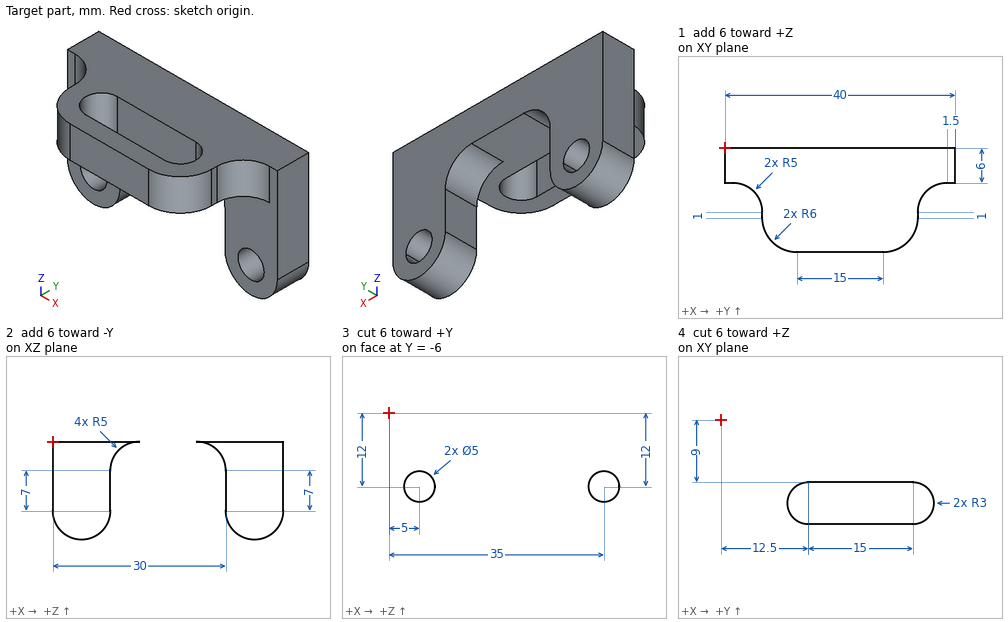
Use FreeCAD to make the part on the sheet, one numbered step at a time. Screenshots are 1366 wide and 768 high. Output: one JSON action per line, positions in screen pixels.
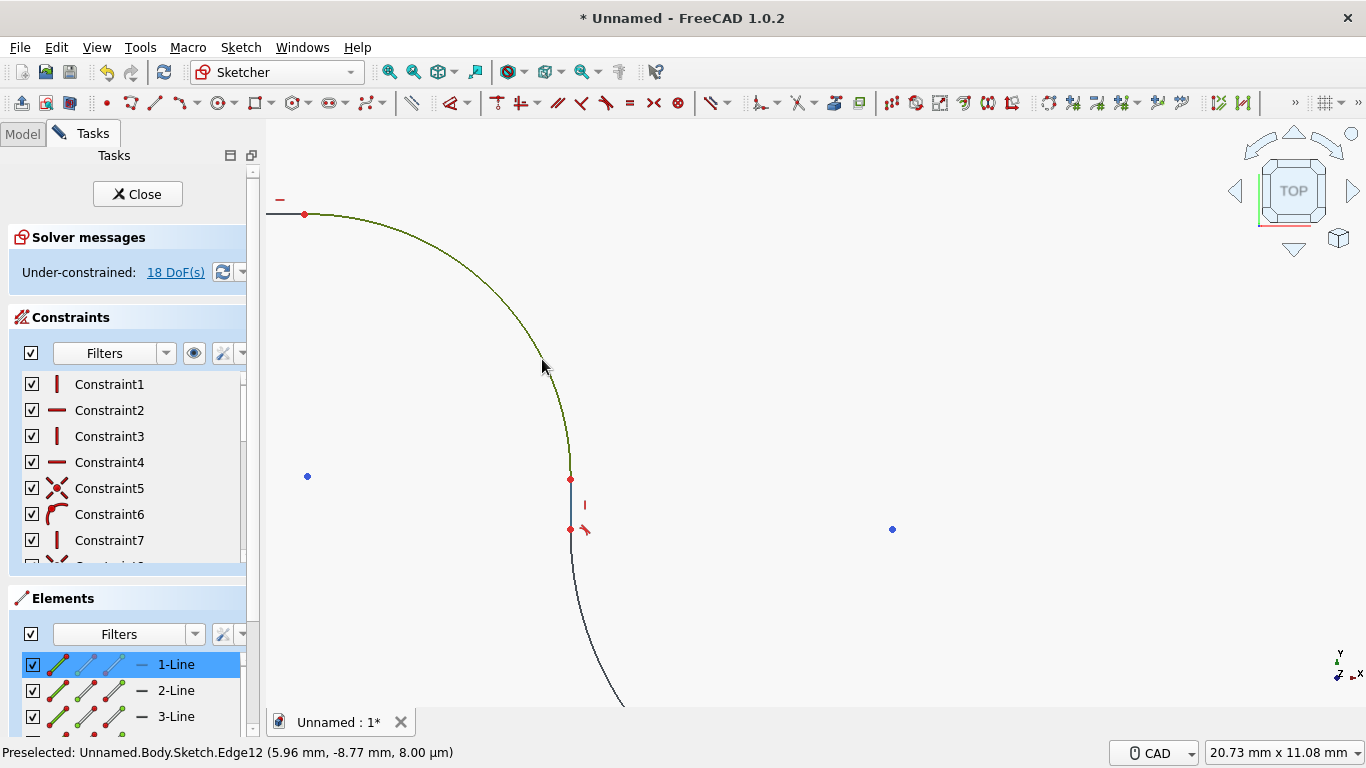
{"action": "key", "text": "t"}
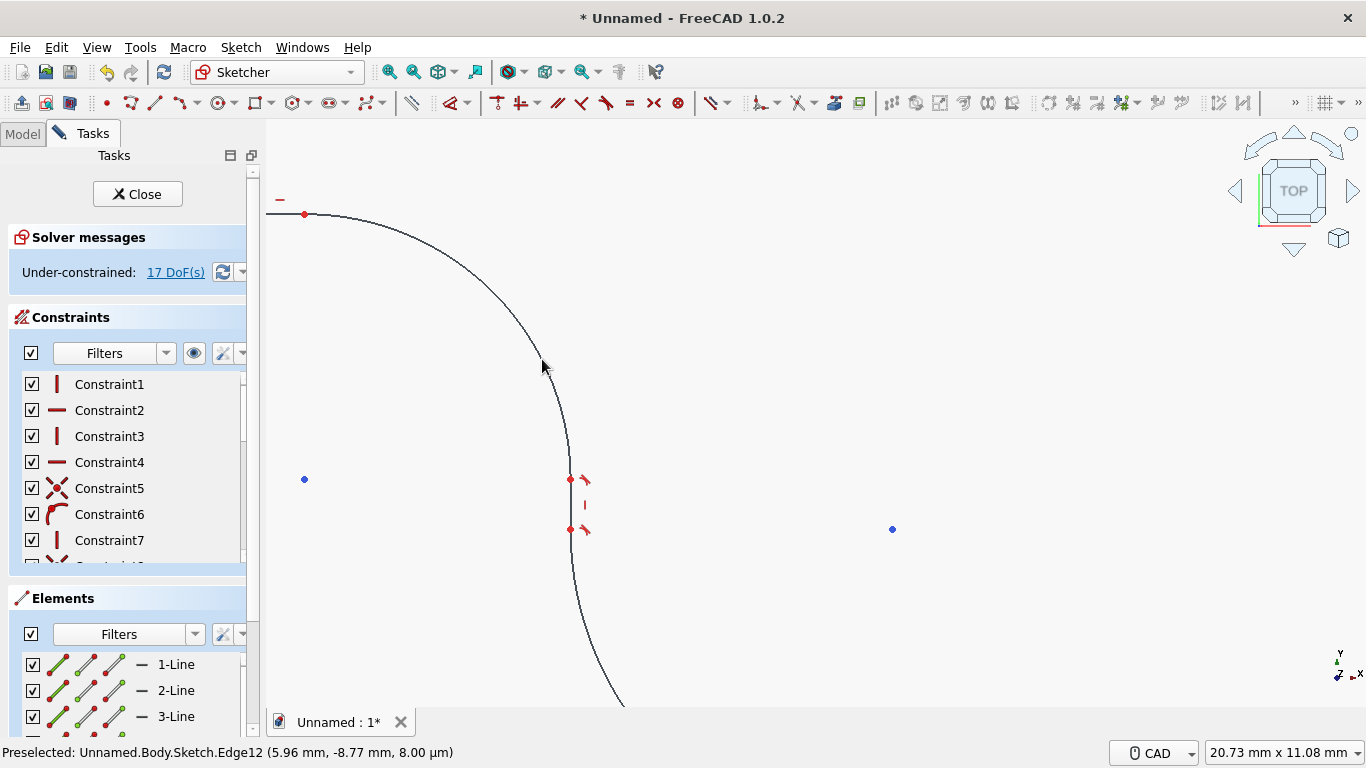
{"action": "scroll", "coordinate": [514, 431], "scroll_direction": "down", "scroll_amount": 6}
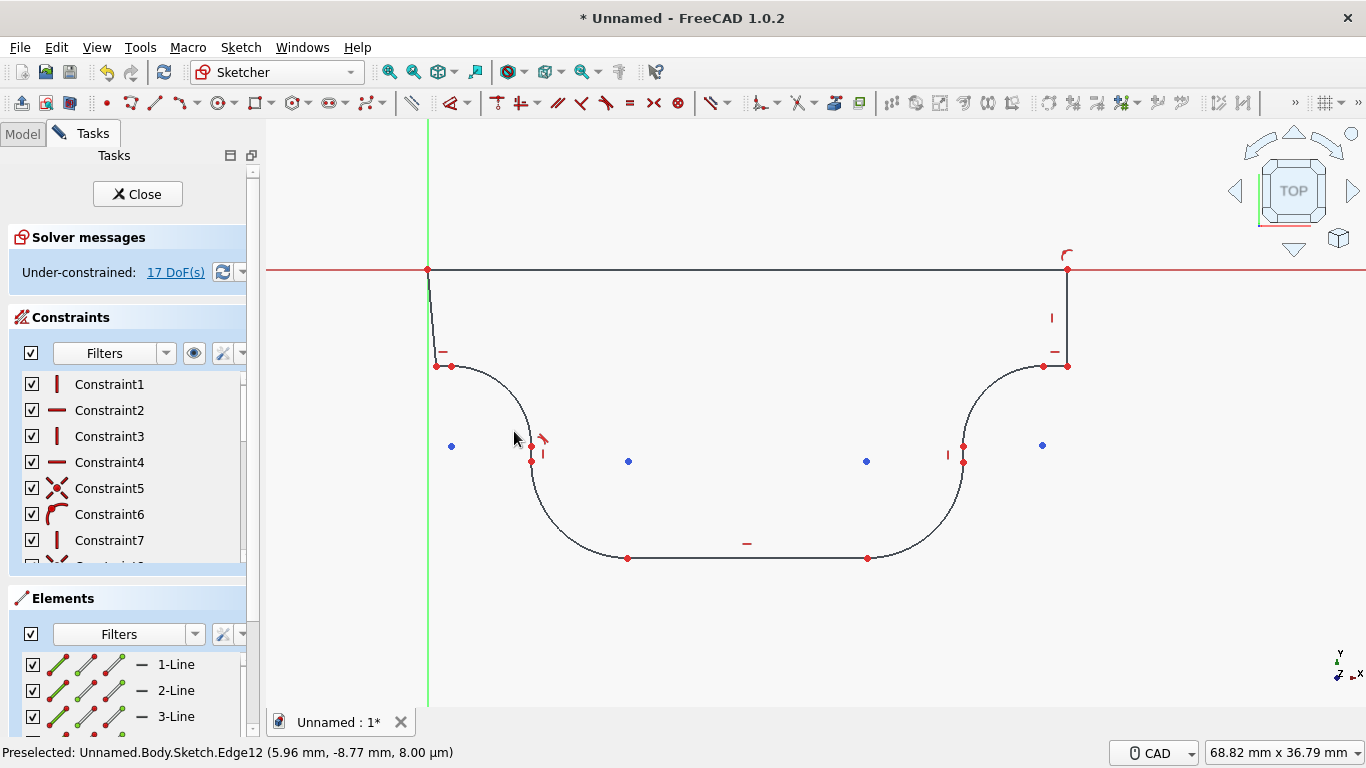
{"action": "left_click", "coordinate": [699, 558]}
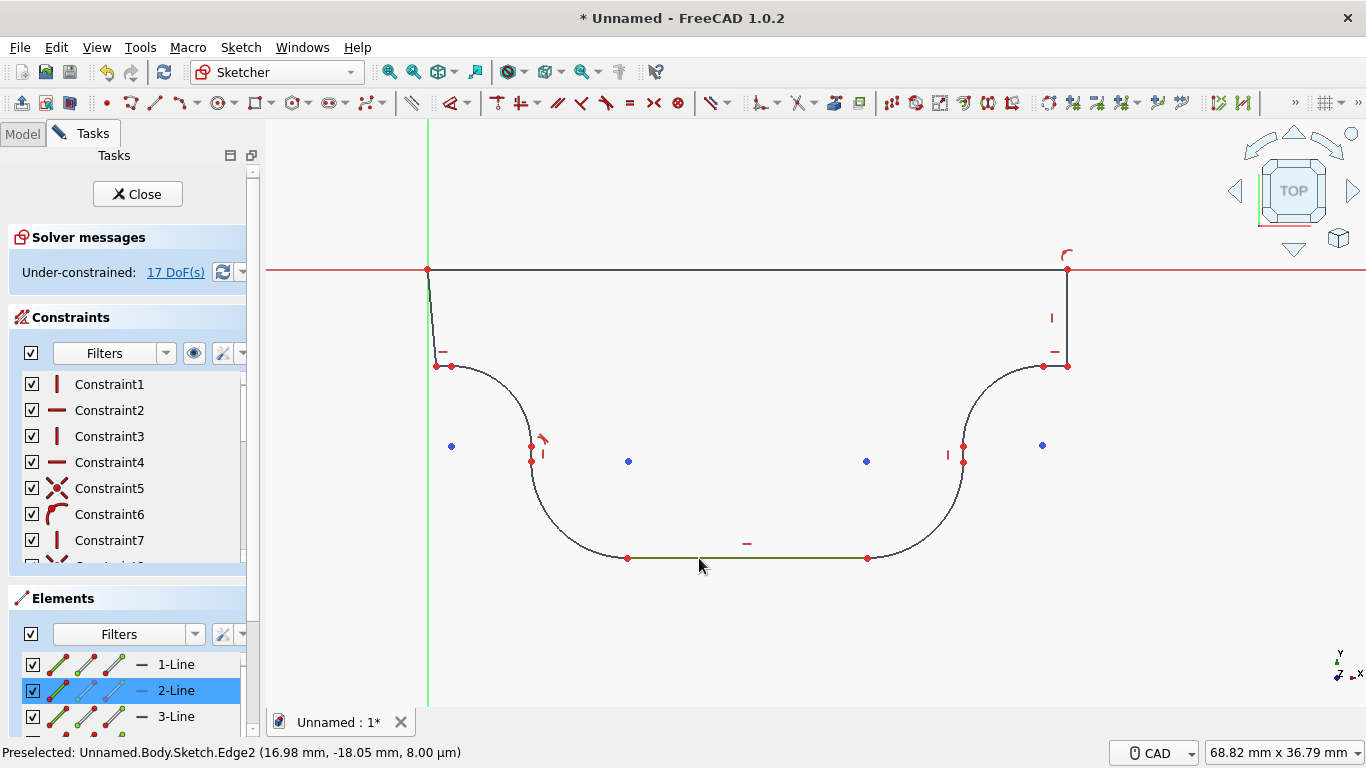
{"action": "left_click", "coordinate": [542, 505]}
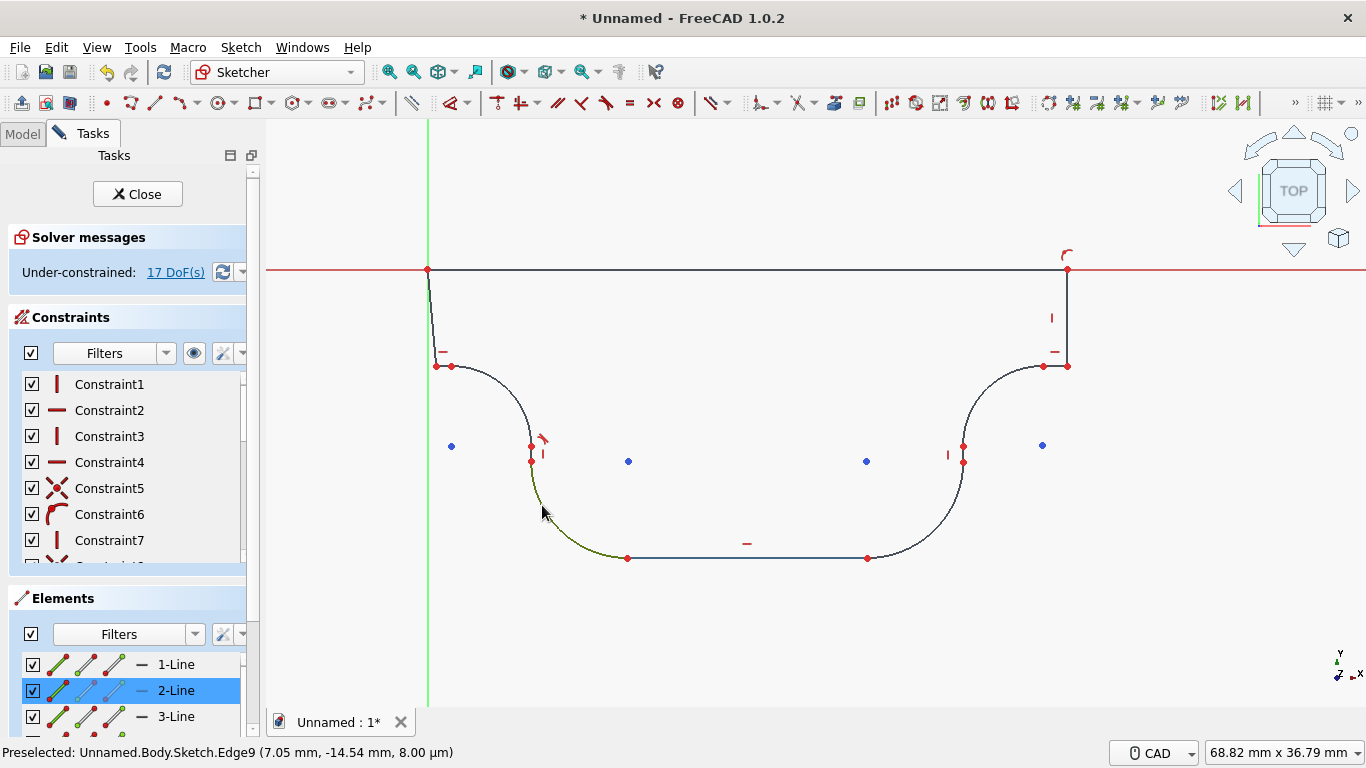
{"action": "key", "text": "t"}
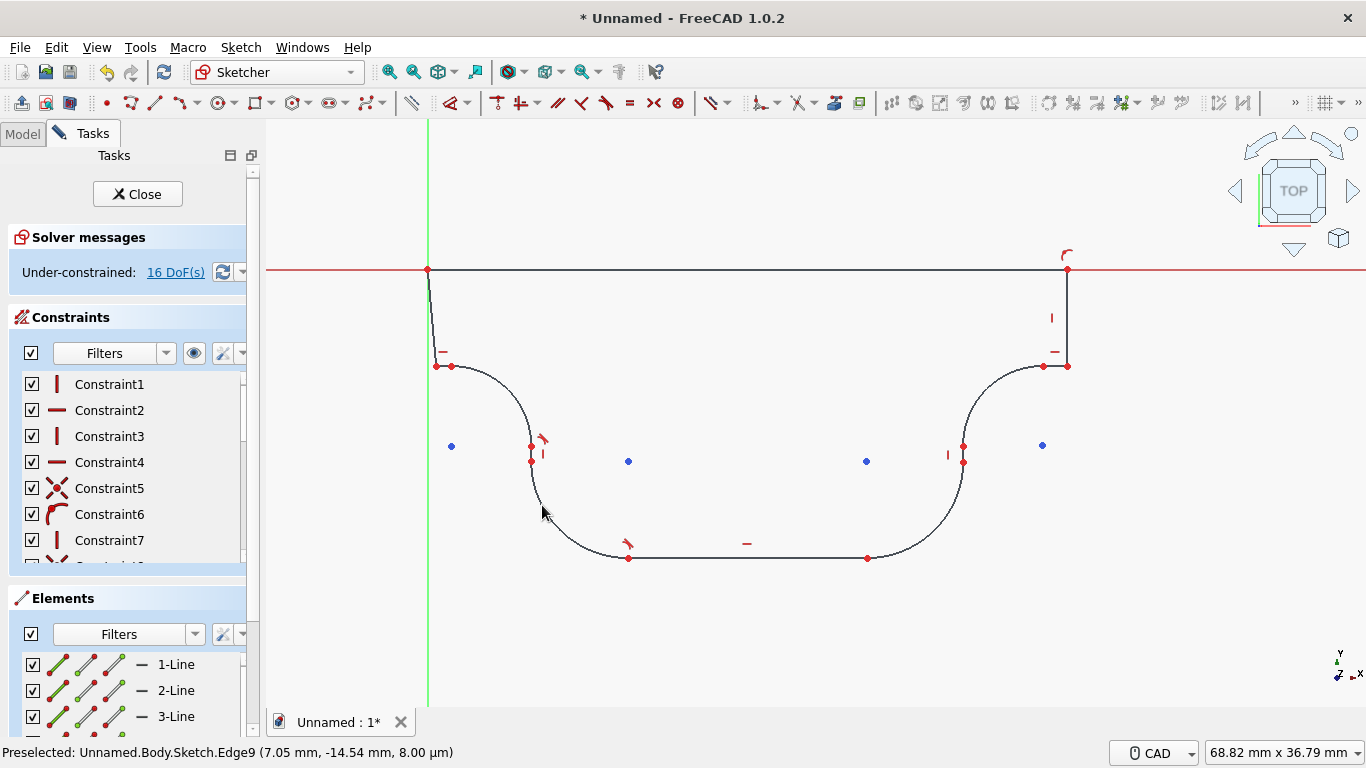
{"action": "left_click", "coordinate": [700, 558]}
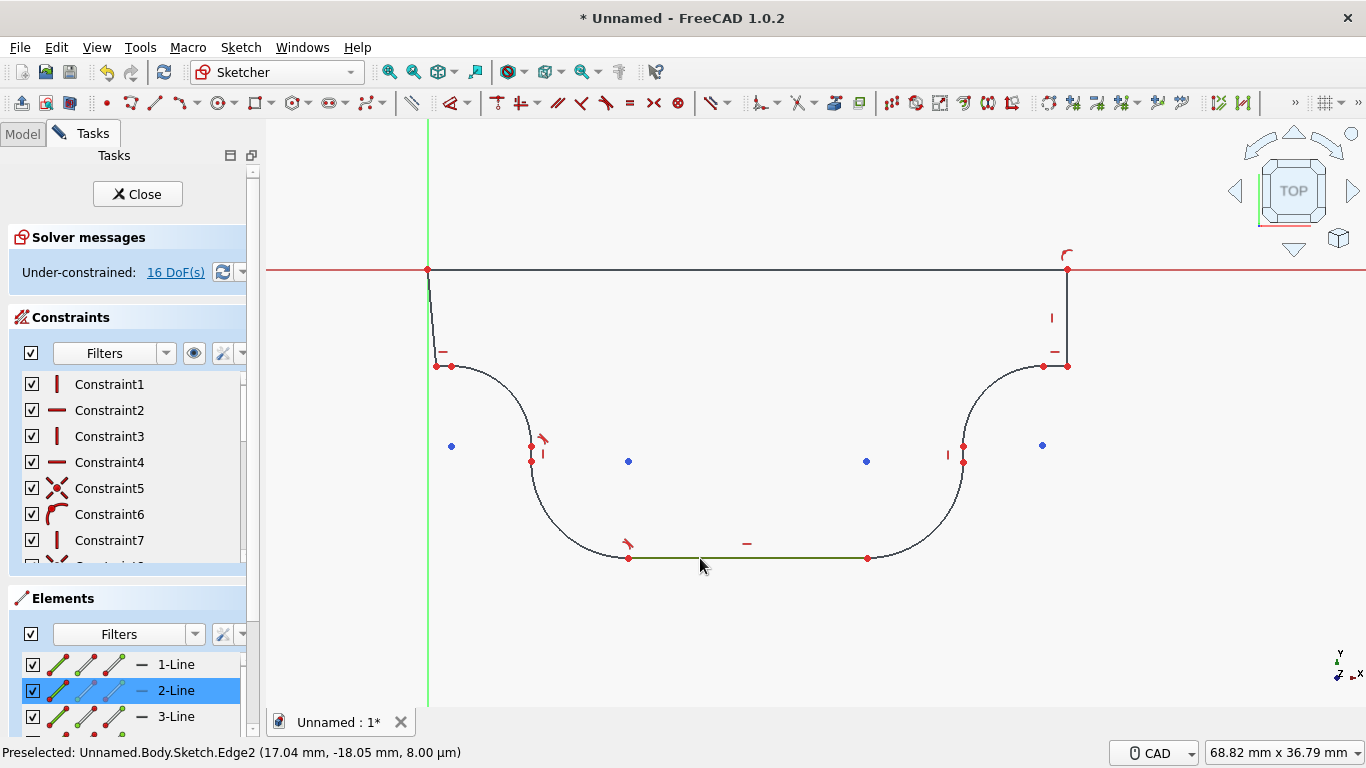
{"action": "left_click", "coordinate": [911, 547]}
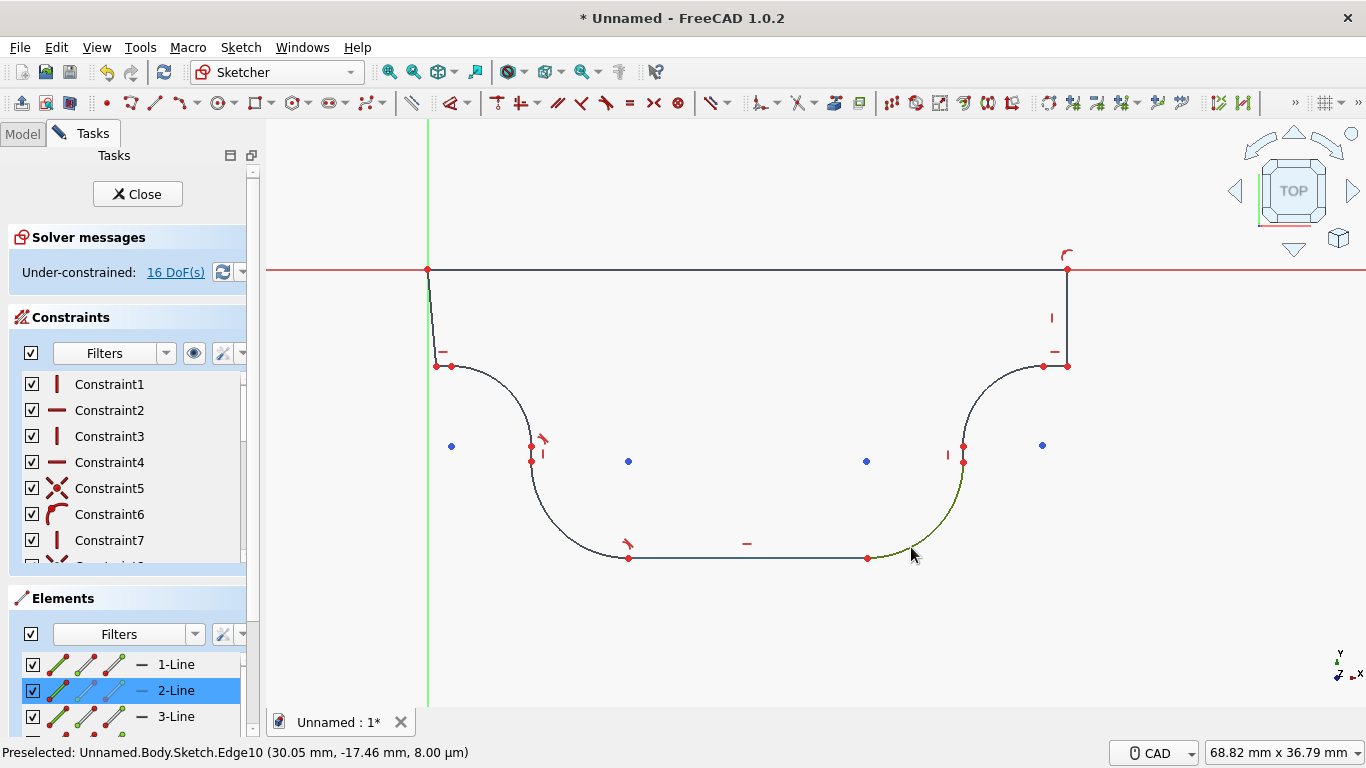
{"action": "left_click", "coordinate": [606, 104]}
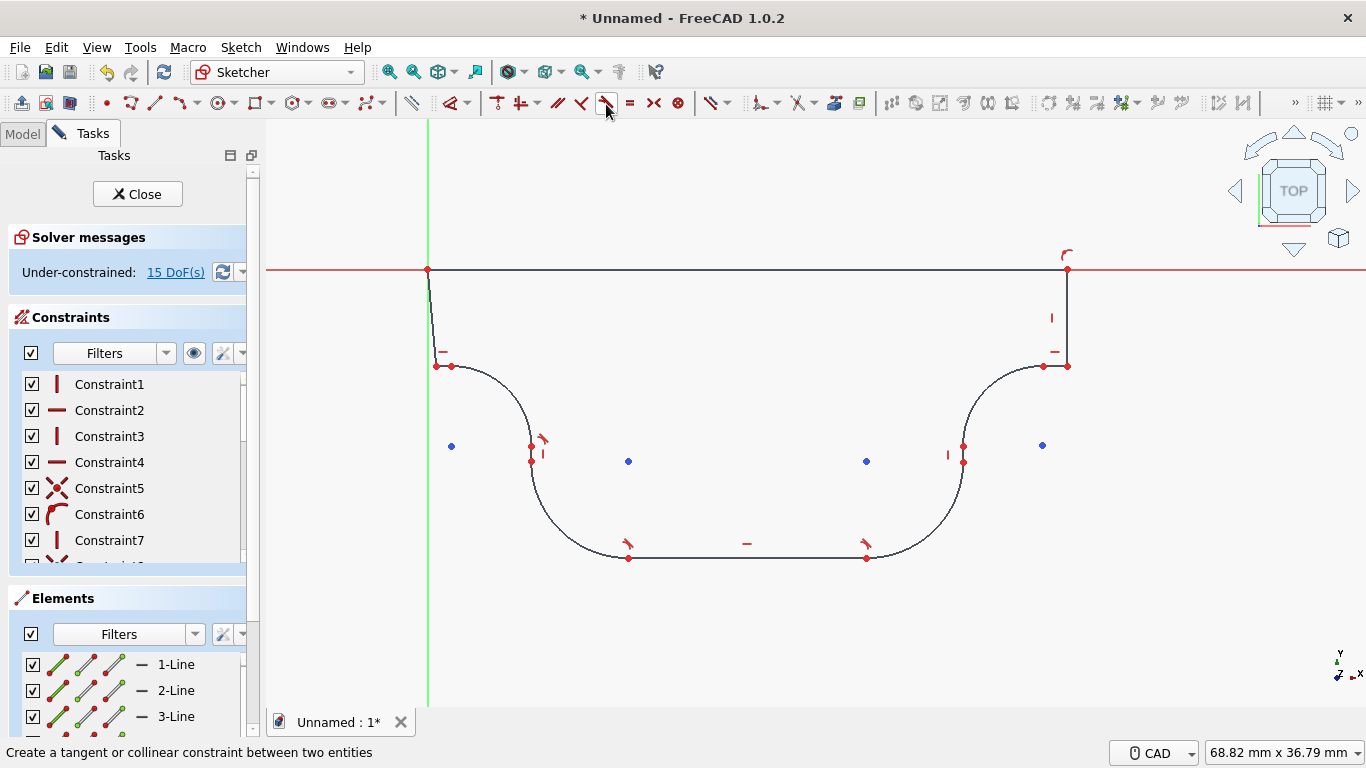
{"action": "scroll", "coordinate": [963, 454], "scroll_direction": "up", "scroll_amount": 3}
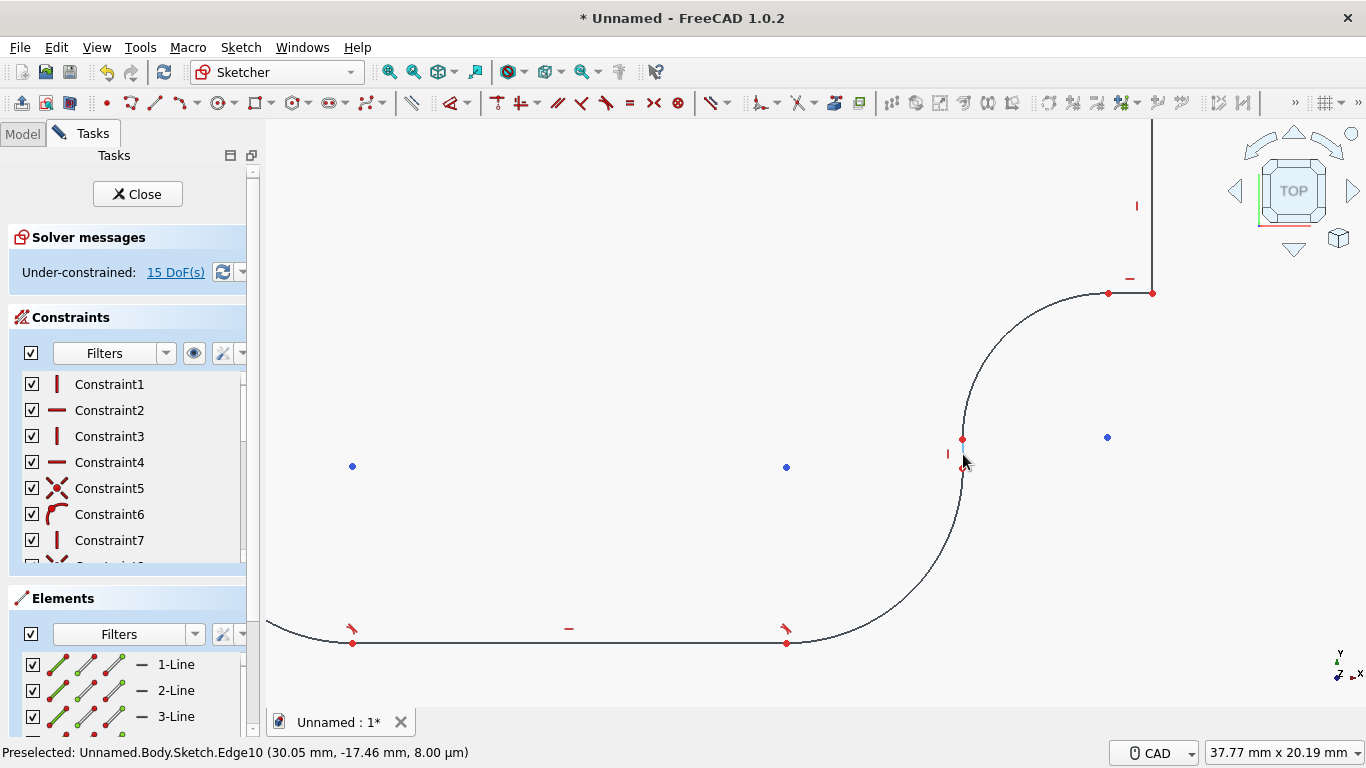
{"action": "left_click", "coordinate": [963, 454]}